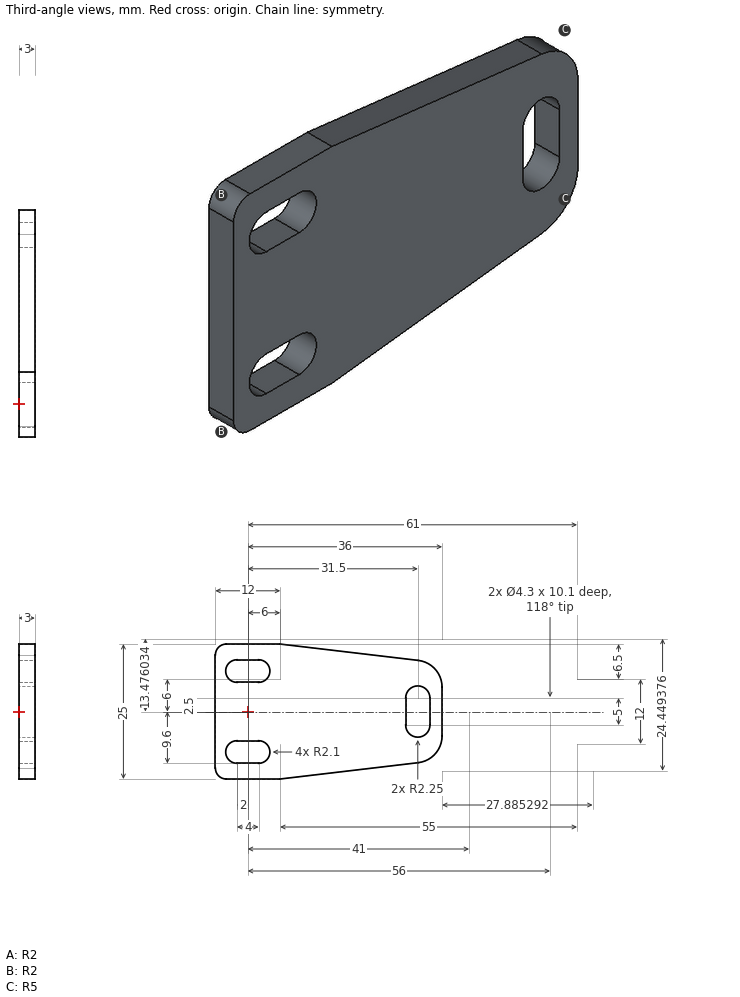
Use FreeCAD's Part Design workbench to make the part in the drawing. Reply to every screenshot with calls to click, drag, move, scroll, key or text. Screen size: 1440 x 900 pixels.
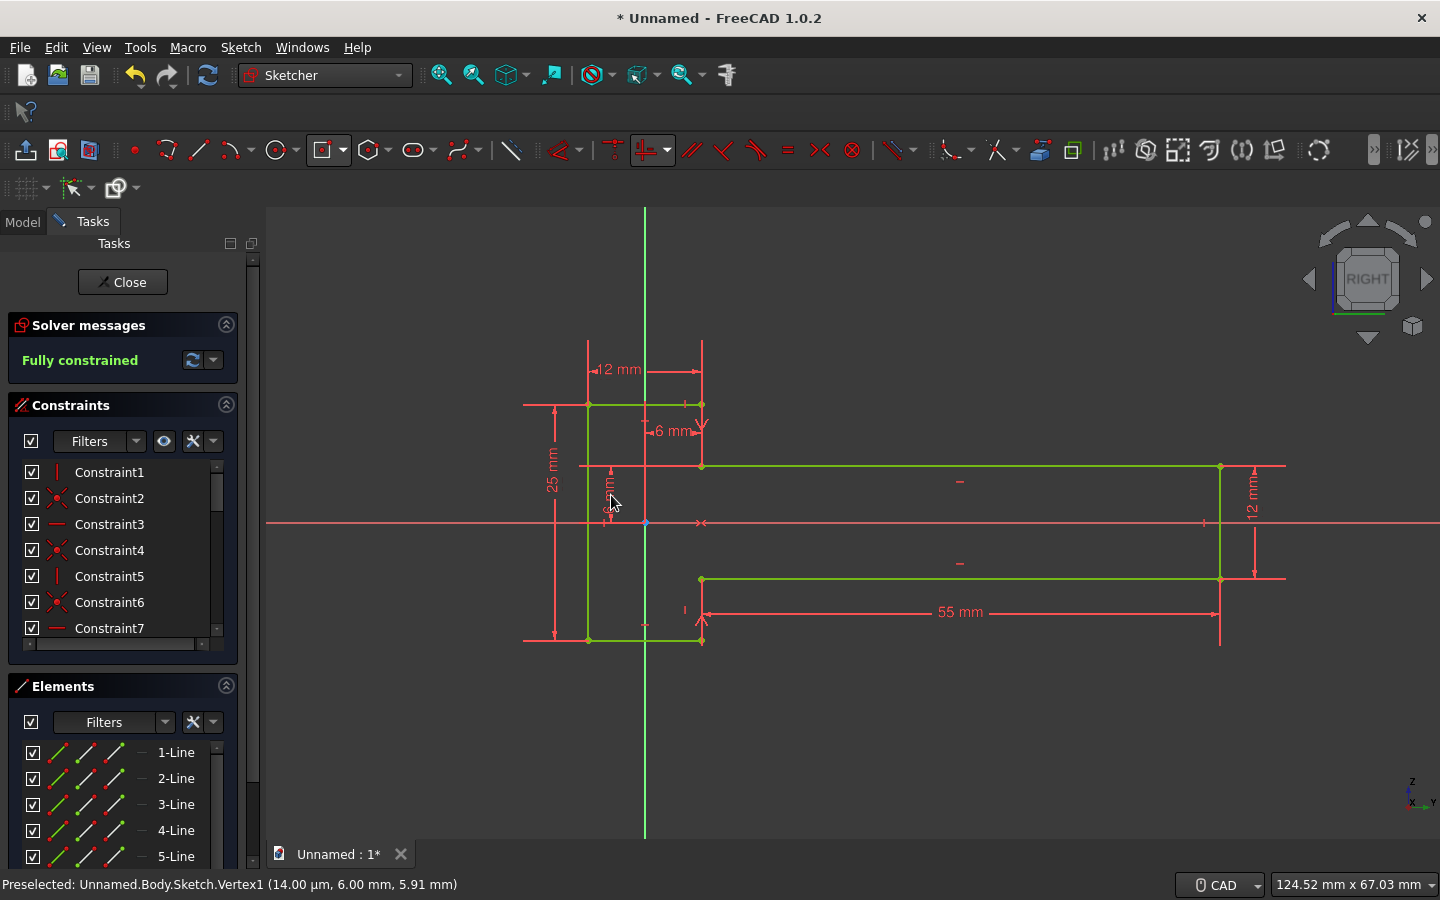
click(123, 282)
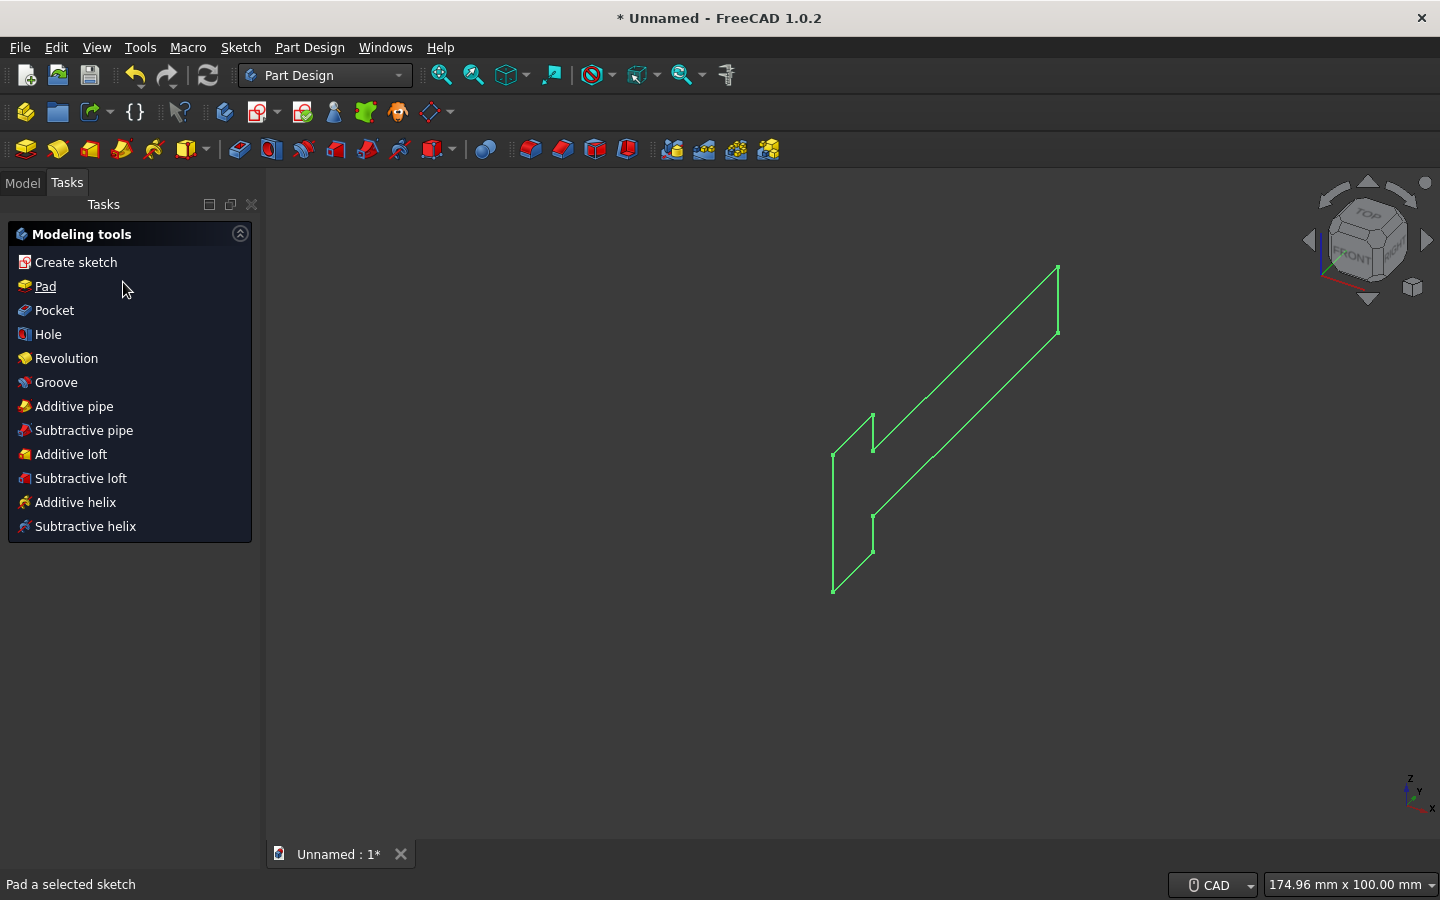
click(26, 150)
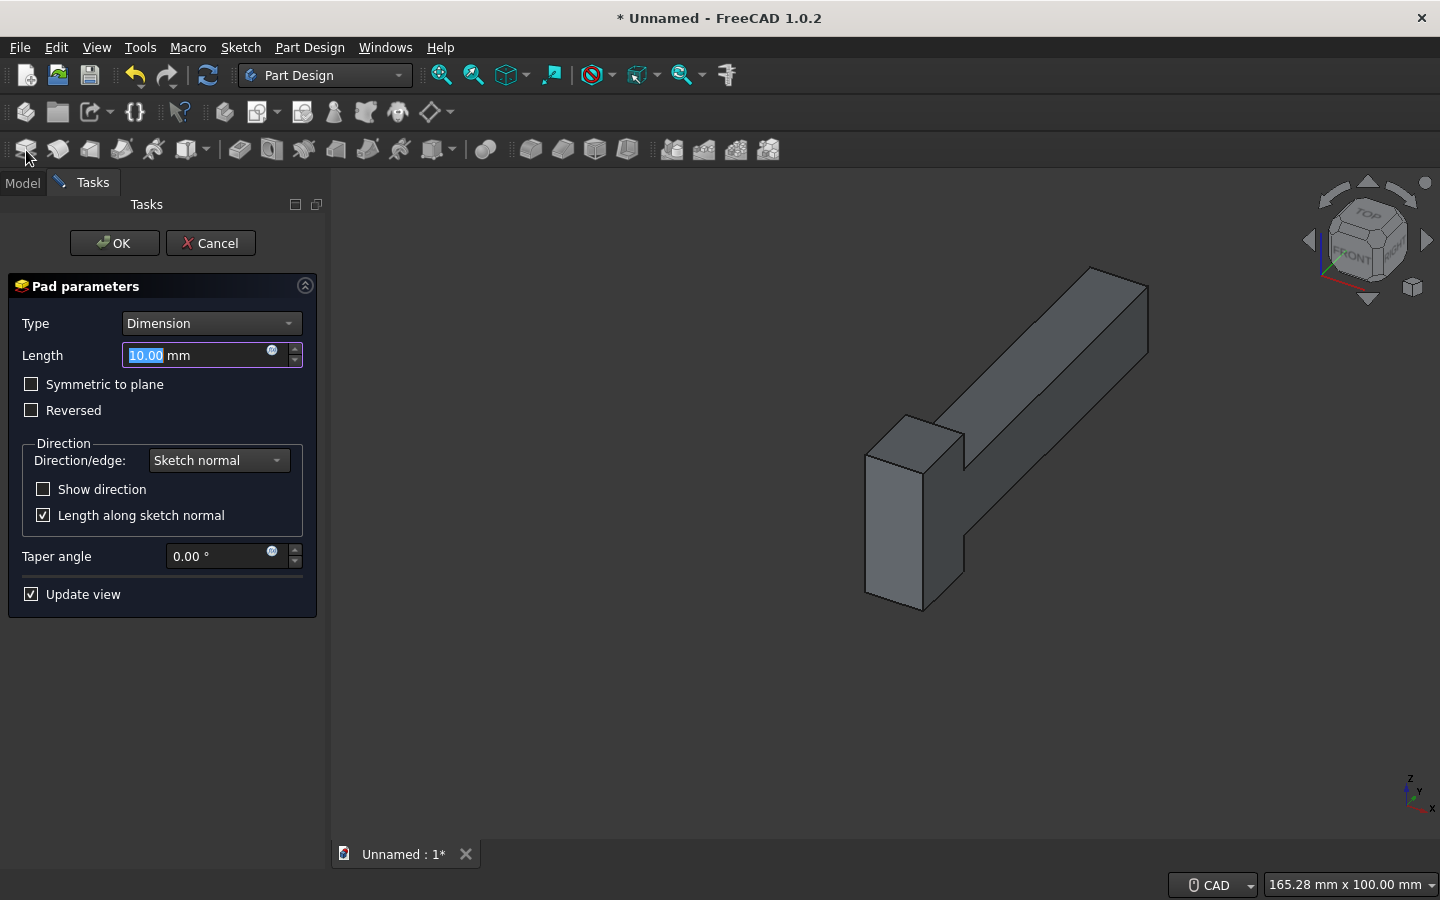
text(3)
key(Tab)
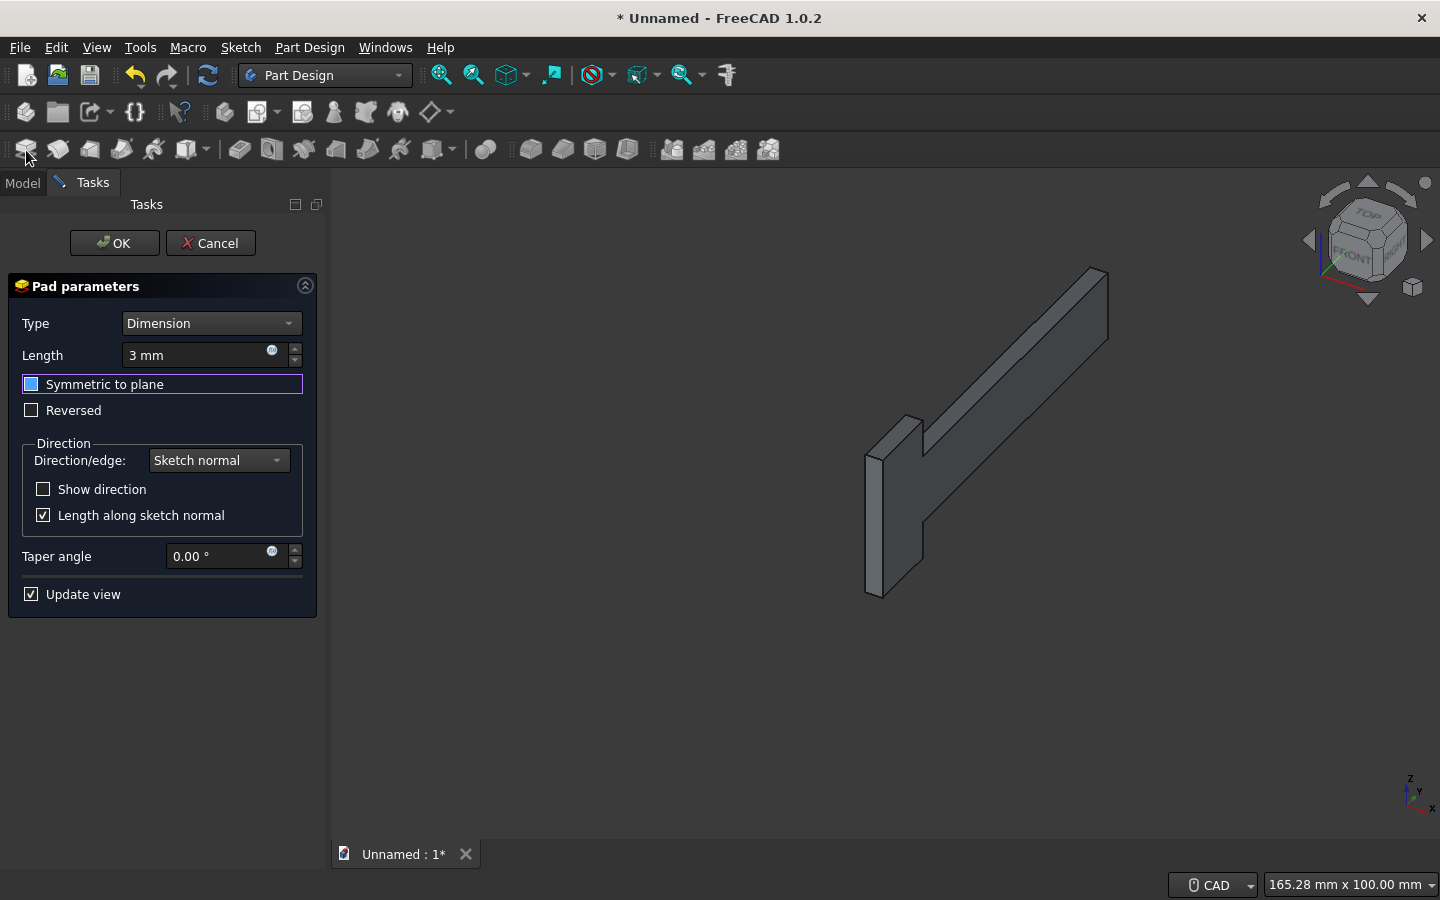
click(115, 243)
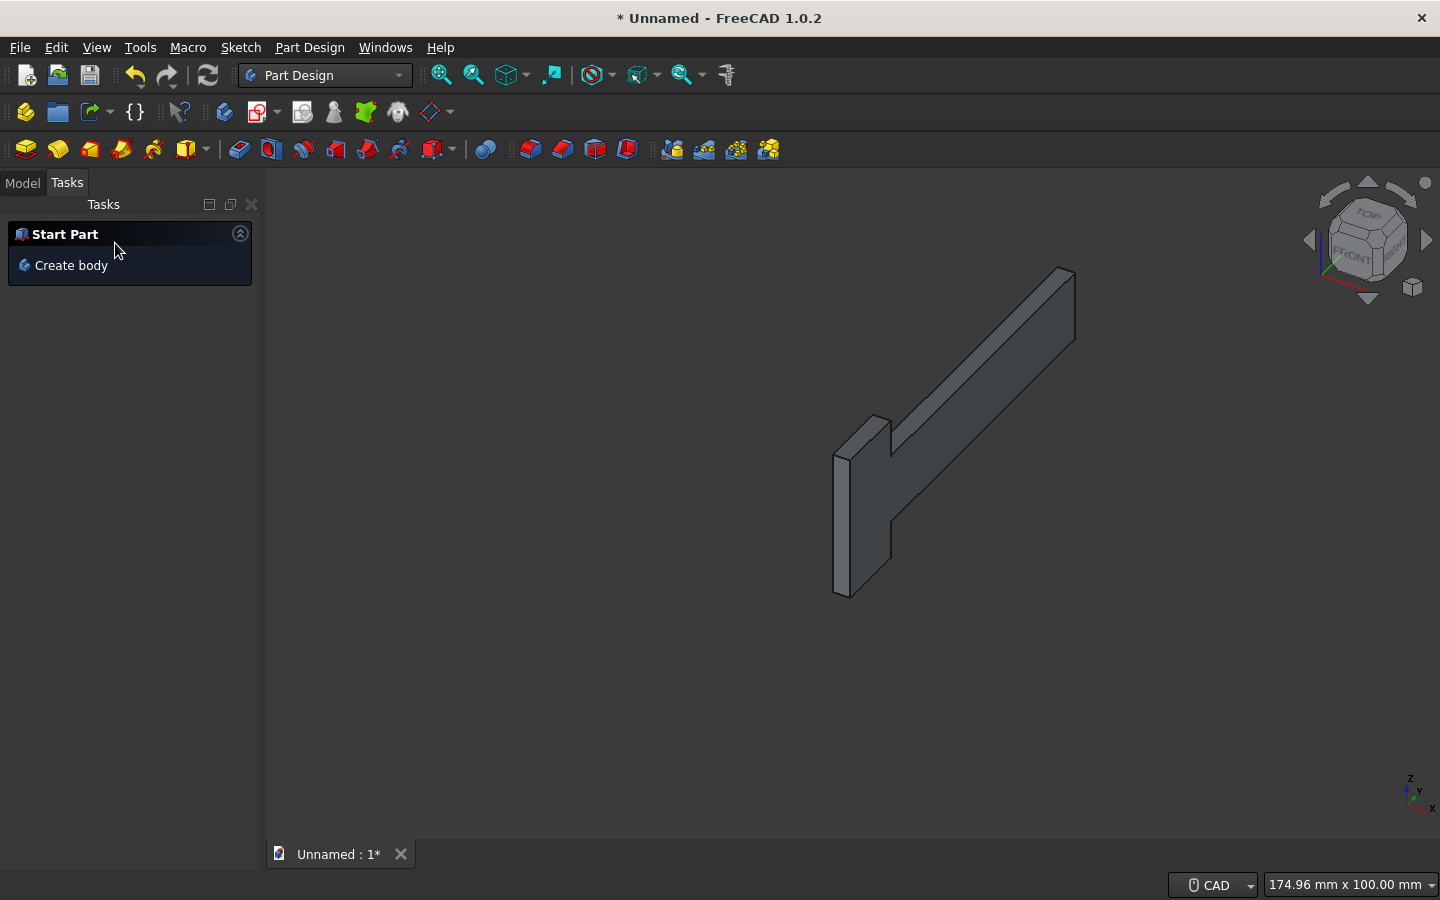
click(258, 112)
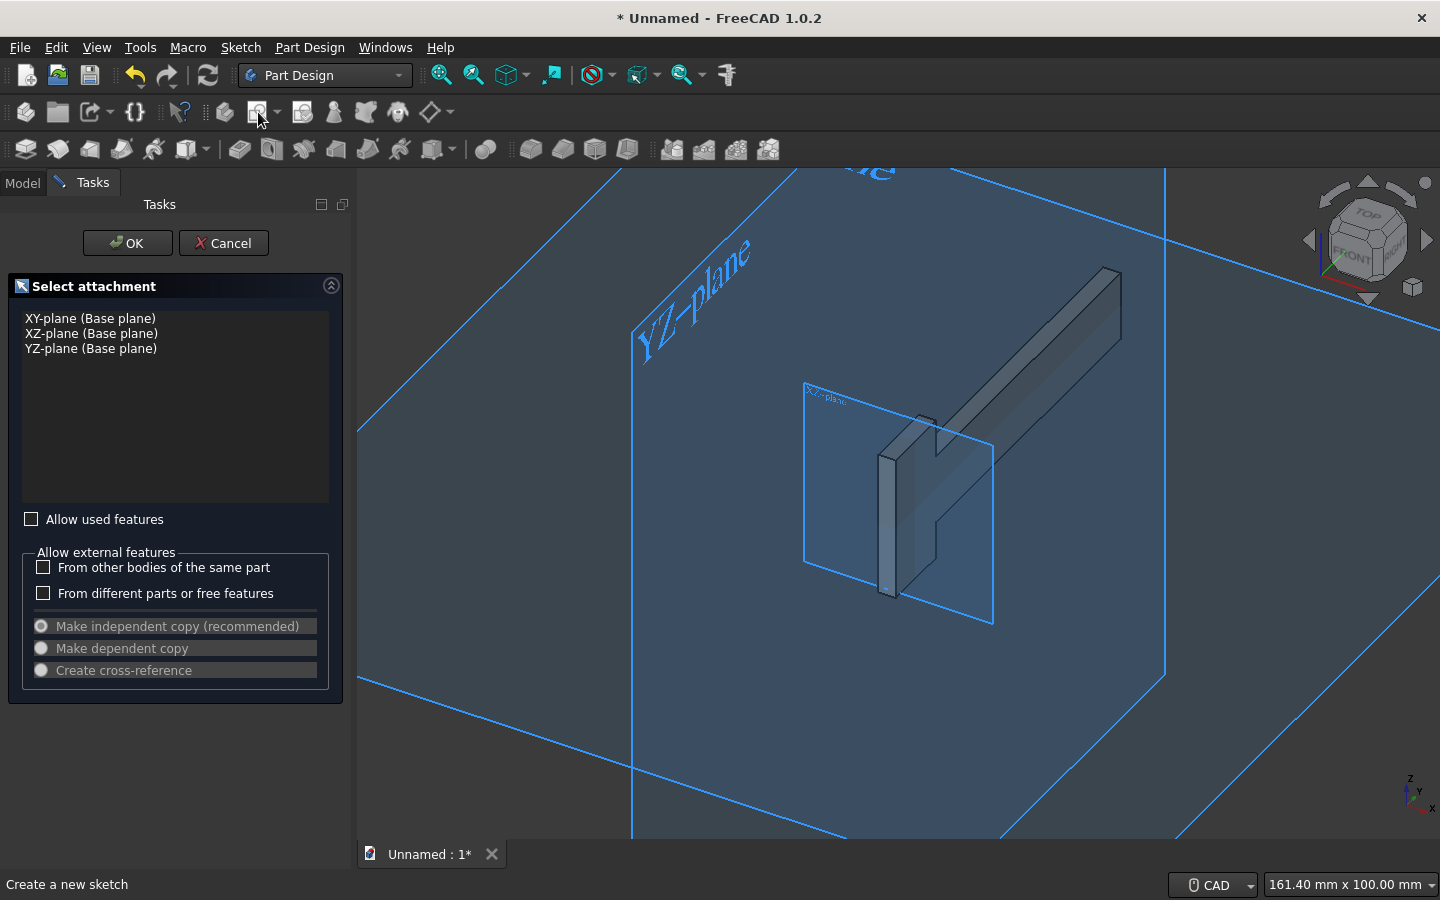
click(82, 348)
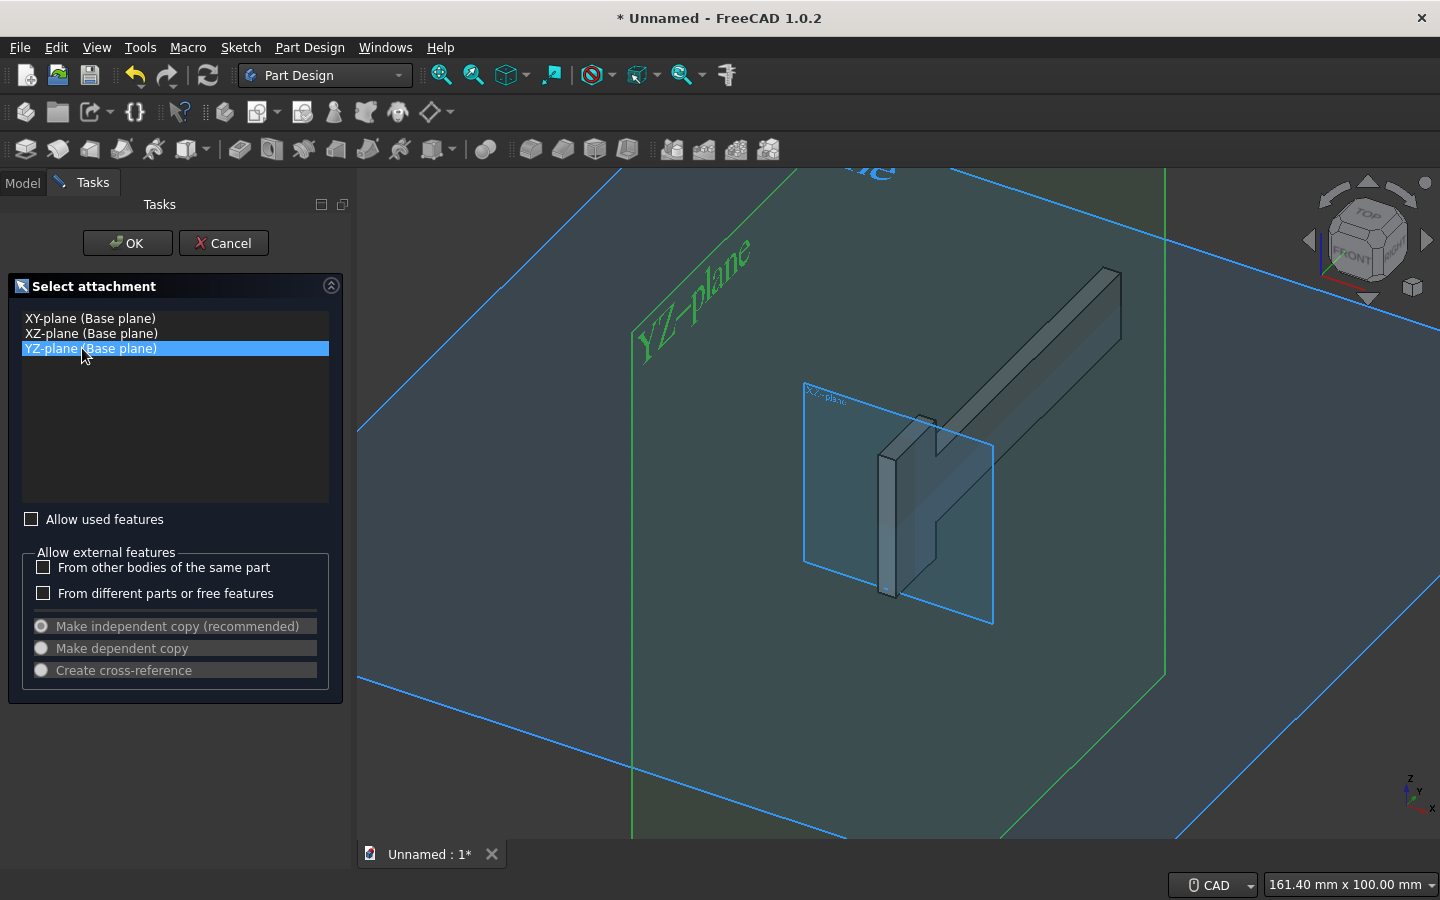
click(128, 243)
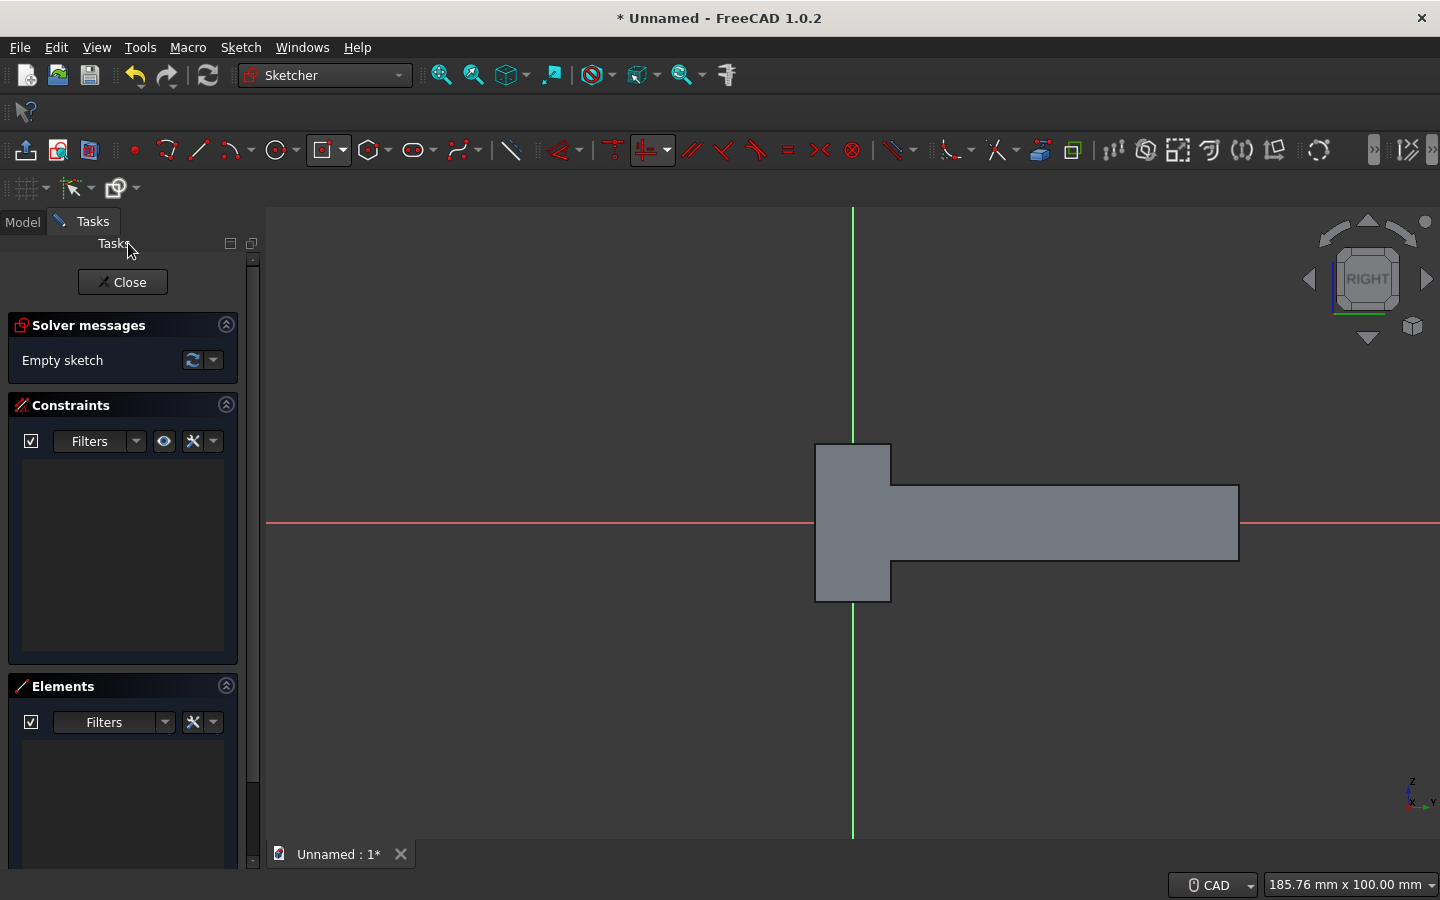
key(q)
key(s)